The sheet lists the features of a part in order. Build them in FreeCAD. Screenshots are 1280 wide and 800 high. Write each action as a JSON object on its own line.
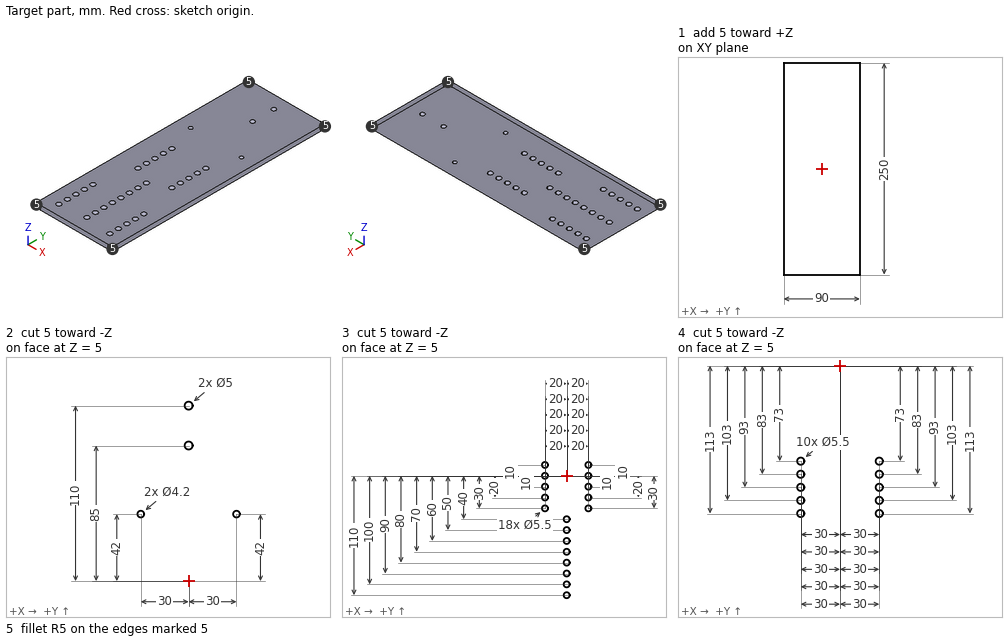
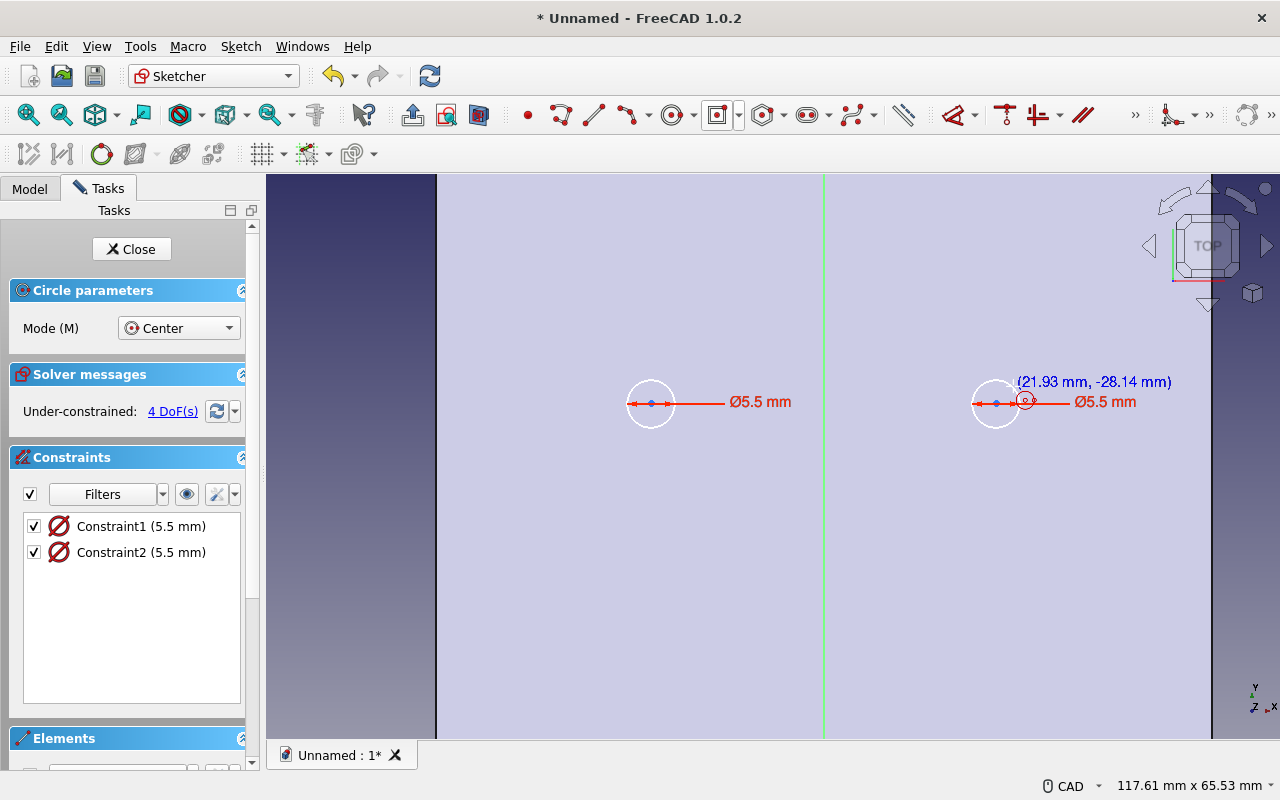
{"action": "scroll", "coordinate": [653, 405], "scroll_direction": "down", "scroll_amount": 6}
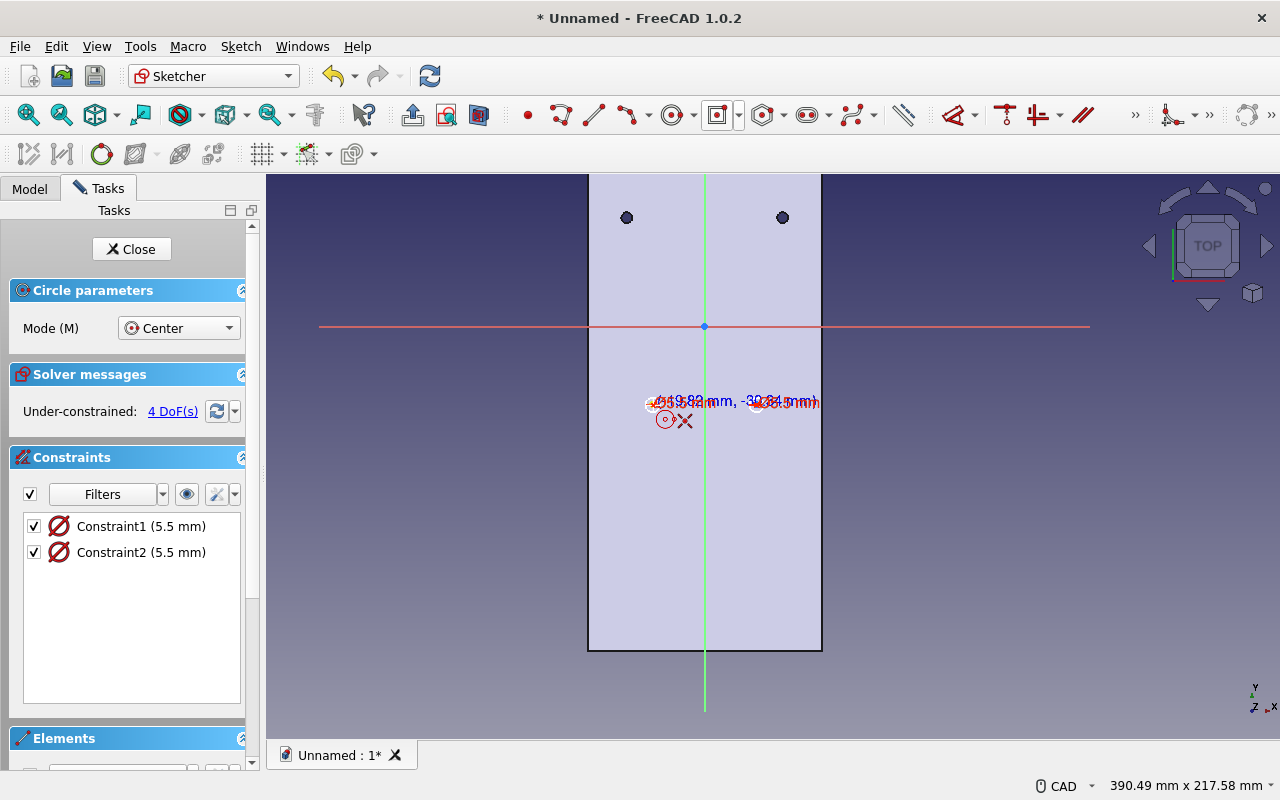
{"action": "scroll", "coordinate": [705, 535], "scroll_direction": "up", "scroll_amount": 6}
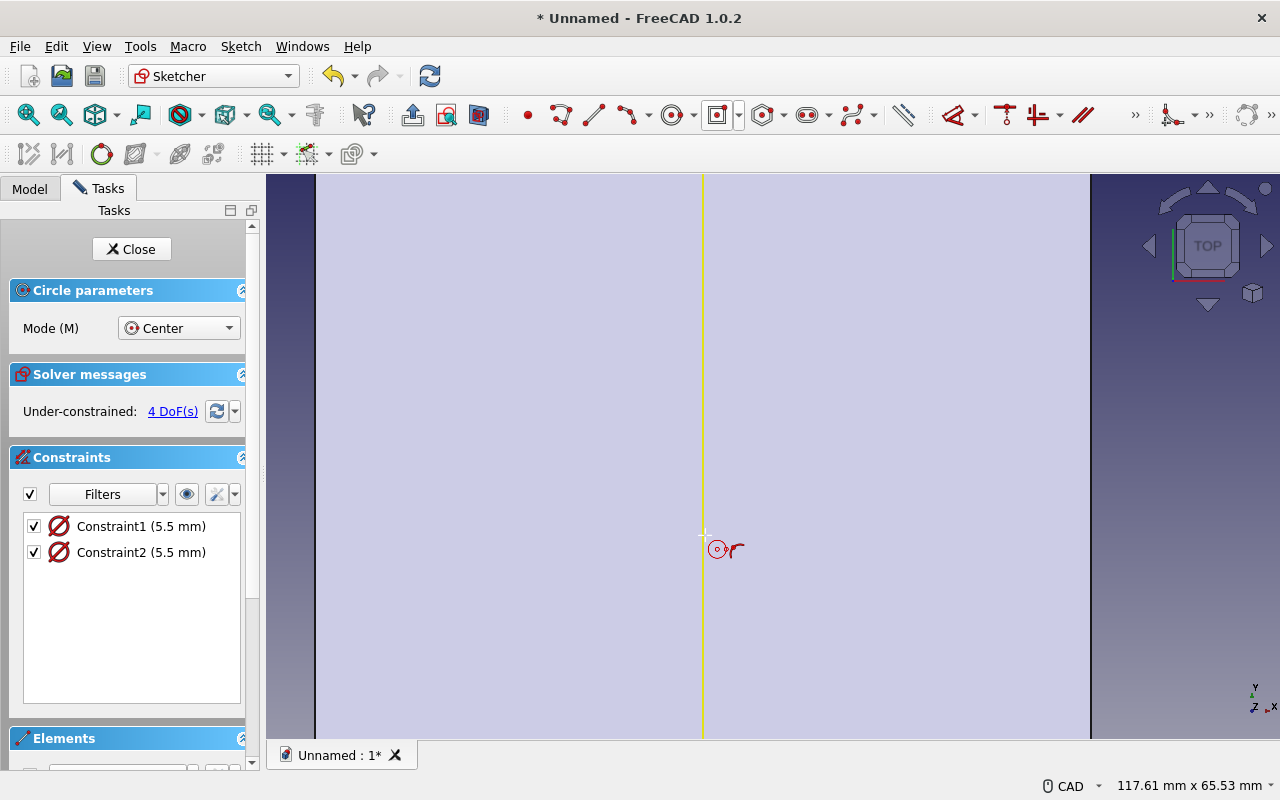
{"action": "left_click", "coordinate": [703, 532]}
{"action": "mouse_move", "coordinate": [720, 515]}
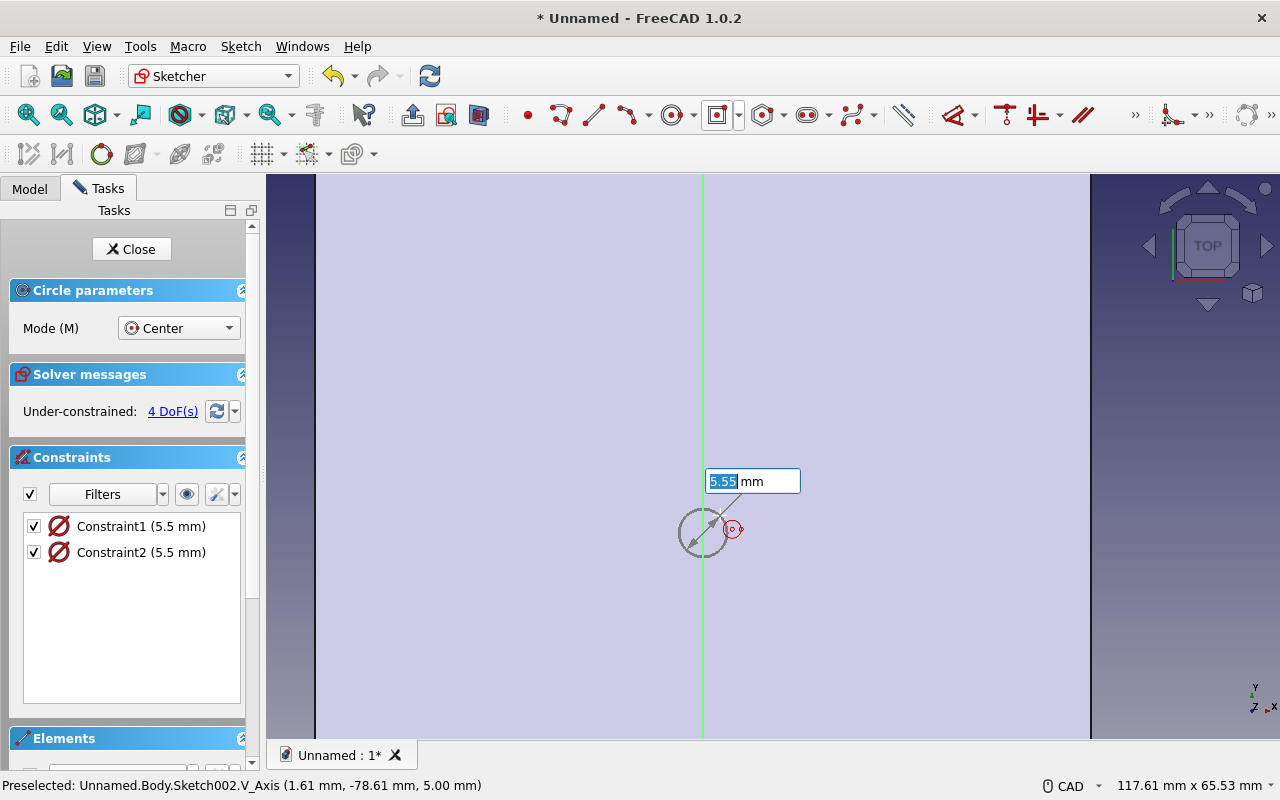
{"action": "type", "text": "5.5"}
{"action": "key", "text": "Return"}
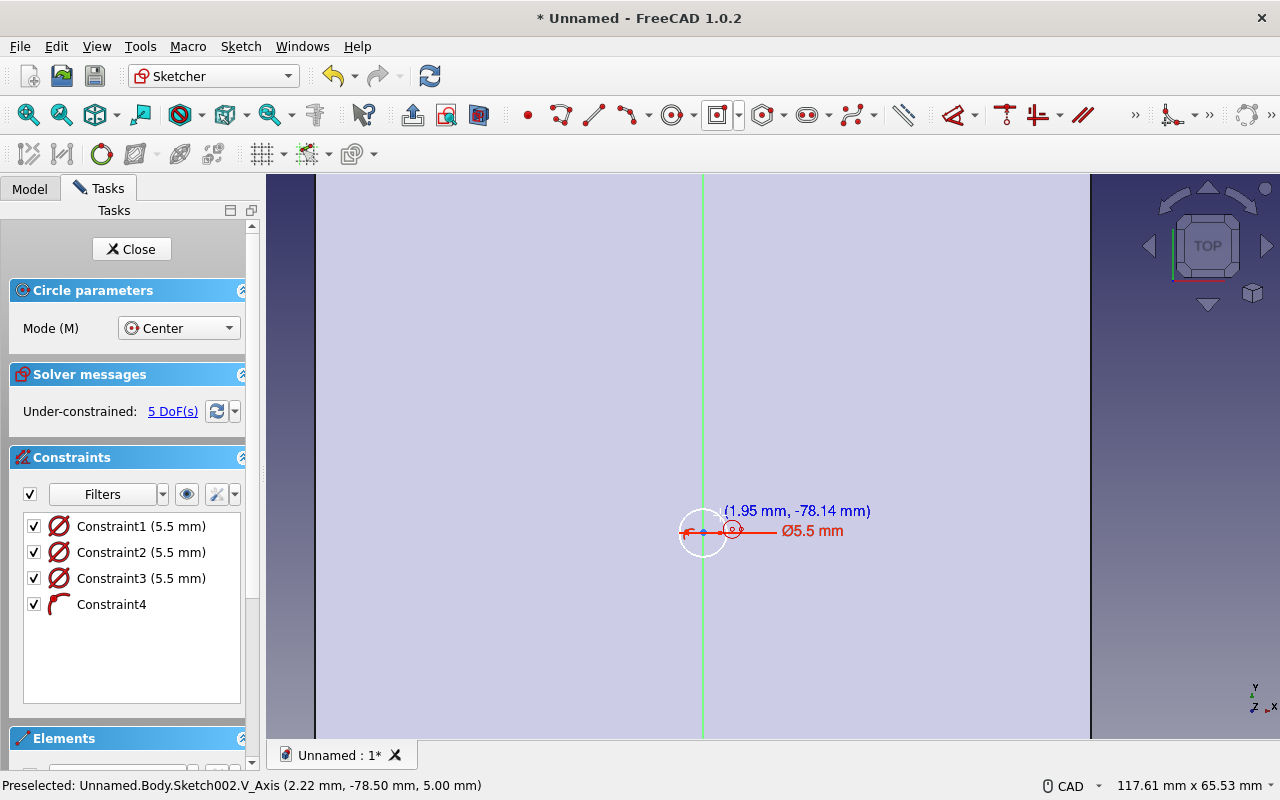
{"action": "left_click", "coordinate": [703, 446]}
{"action": "mouse_move", "coordinate": [720, 429]}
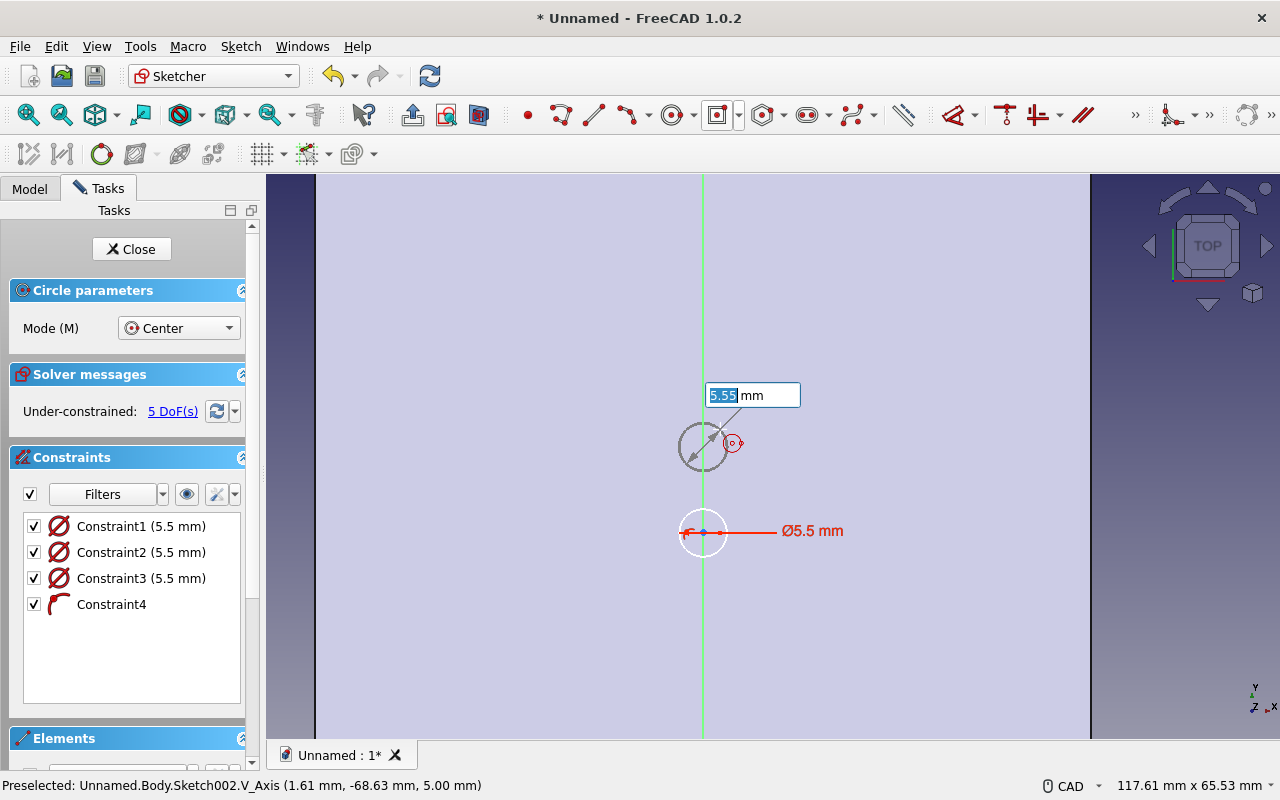
{"action": "type", "text": "5.5"}
{"action": "key", "text": "Return"}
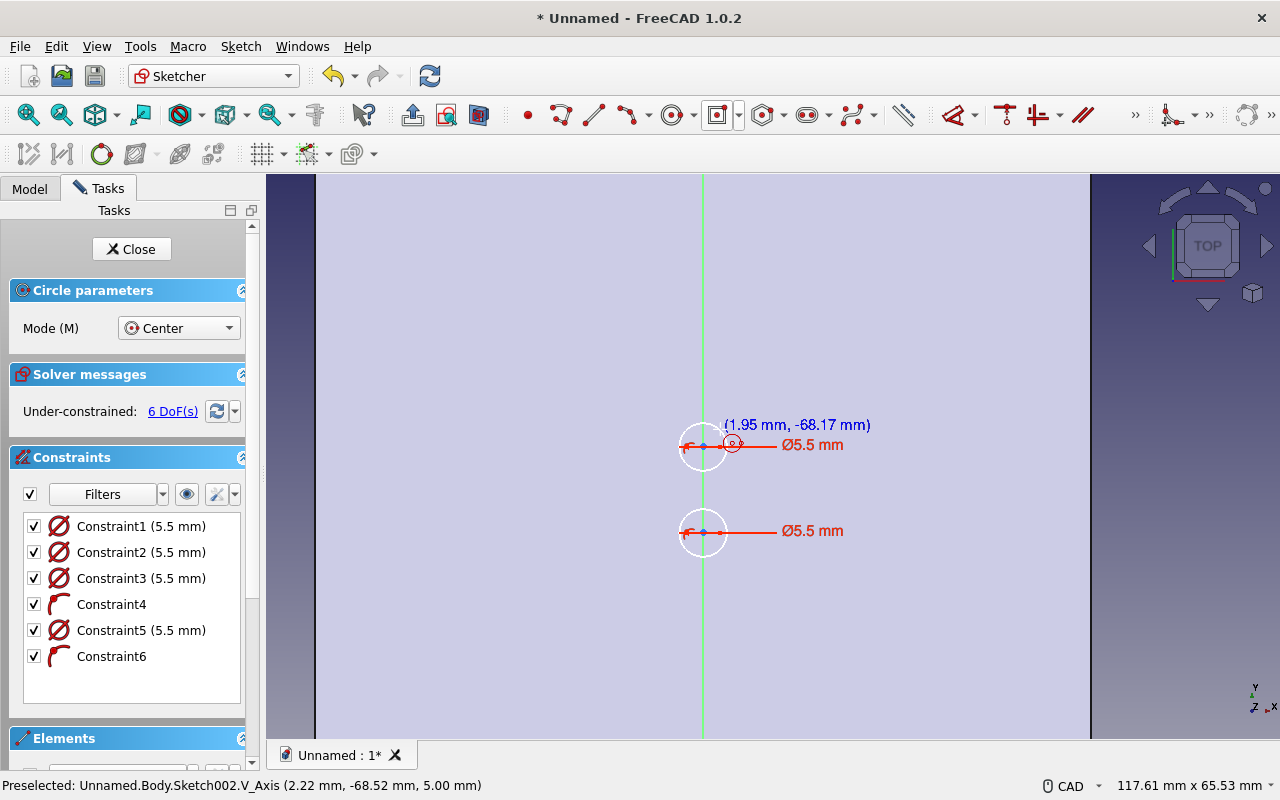
{"action": "left_click", "coordinate": [703, 360]}
{"action": "mouse_move", "coordinate": [720, 343]}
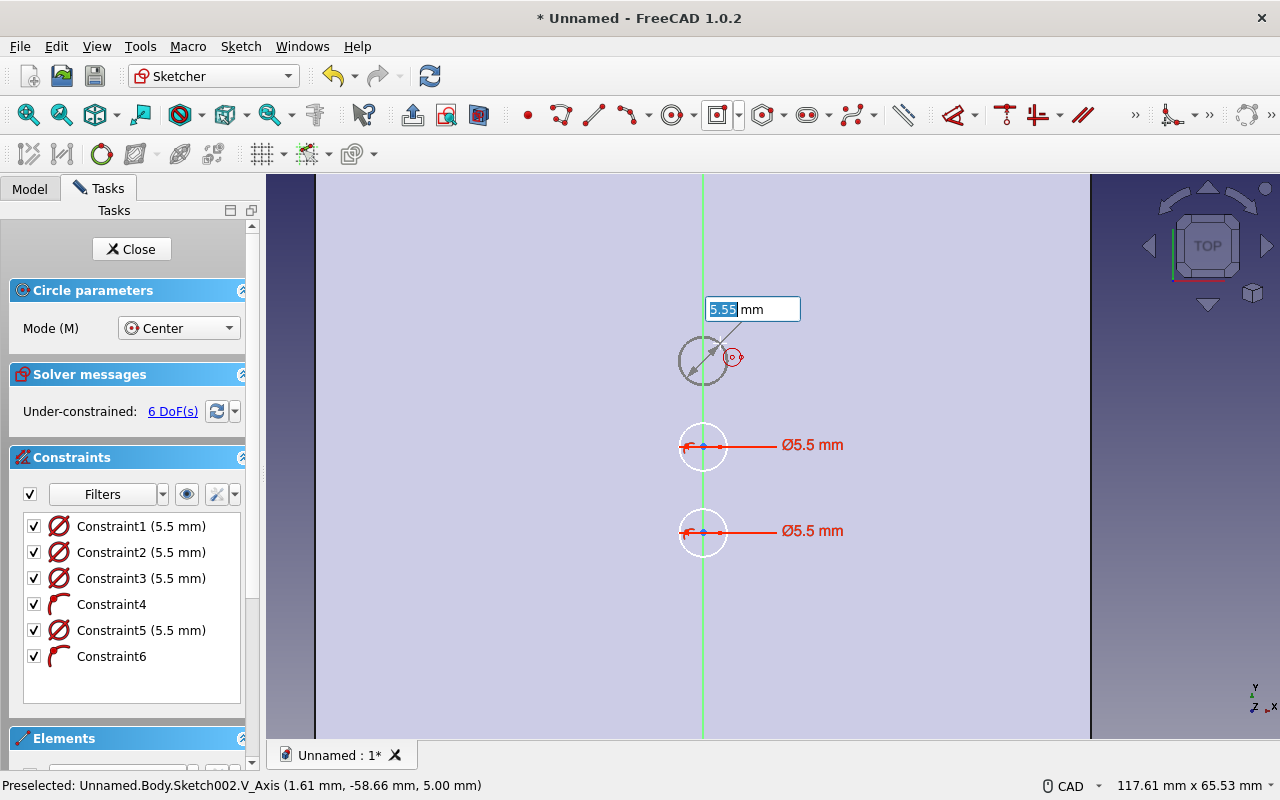
{"action": "type", "text": "5.5"}
{"action": "key", "text": "Return"}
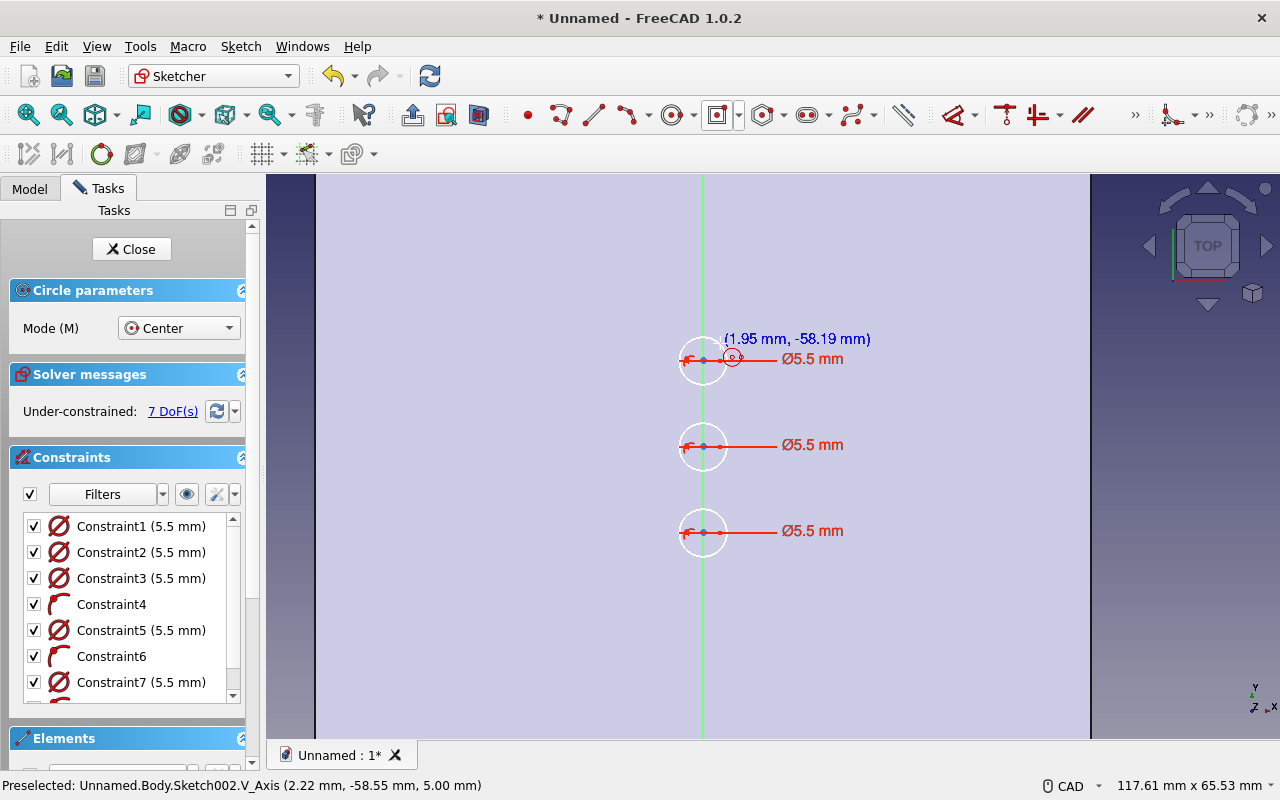
{"action": "left_click", "coordinate": [703, 273]}
{"action": "mouse_move", "coordinate": [720, 257]}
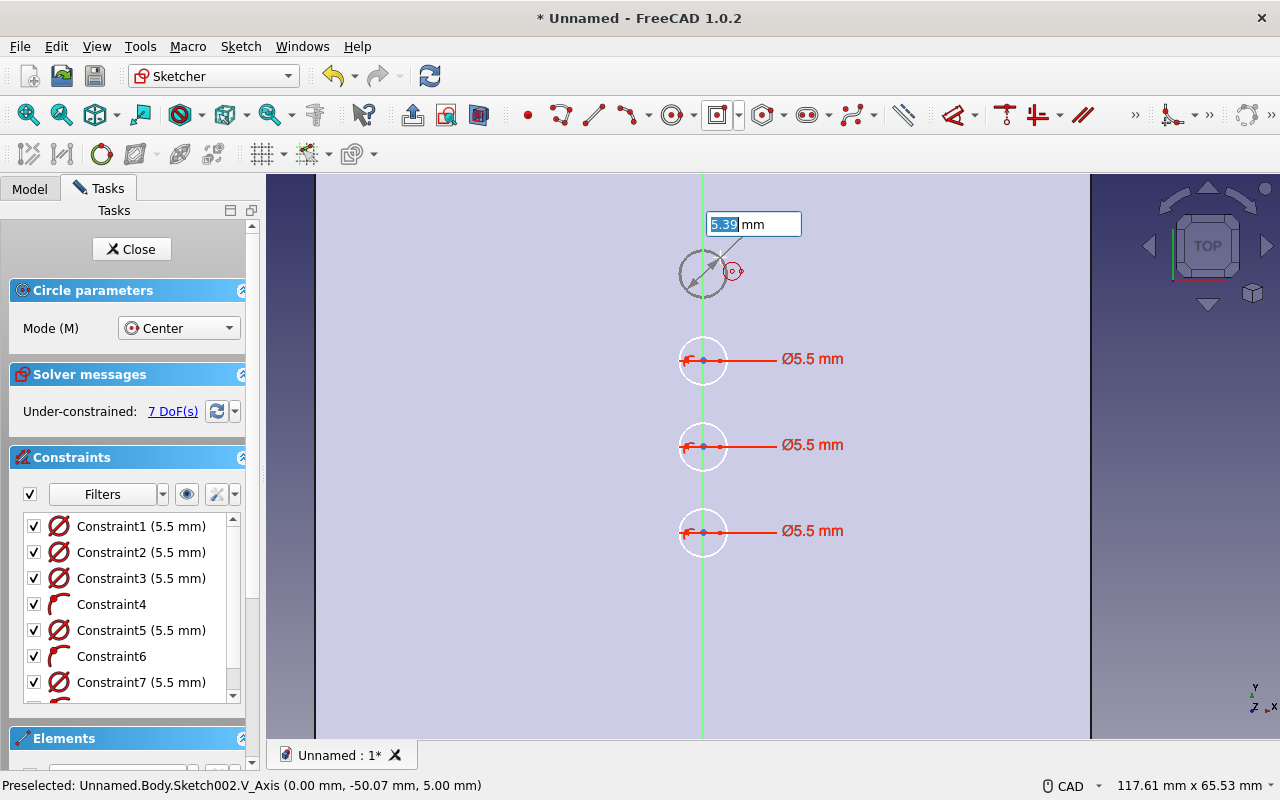
{"action": "type", "text": "5.5"}
{"action": "key", "text": "Return"}